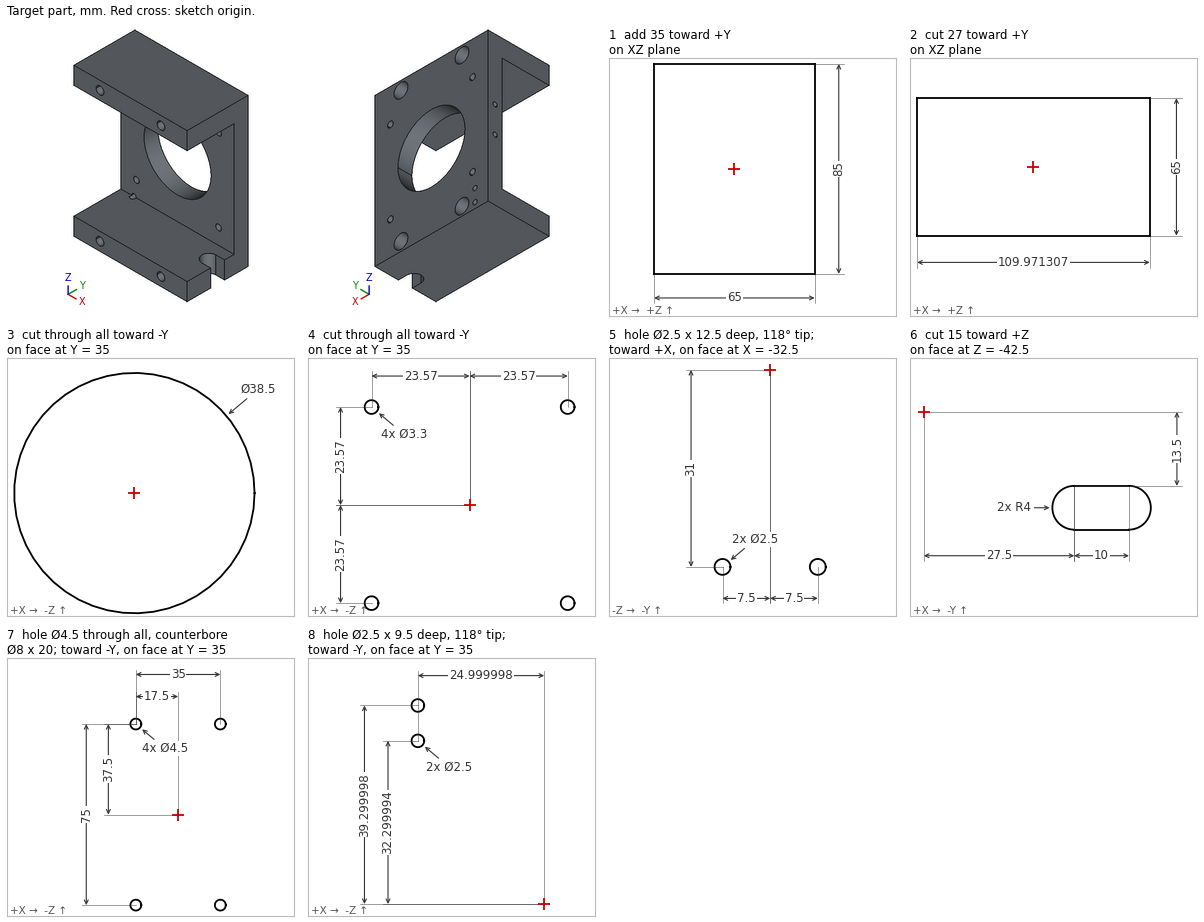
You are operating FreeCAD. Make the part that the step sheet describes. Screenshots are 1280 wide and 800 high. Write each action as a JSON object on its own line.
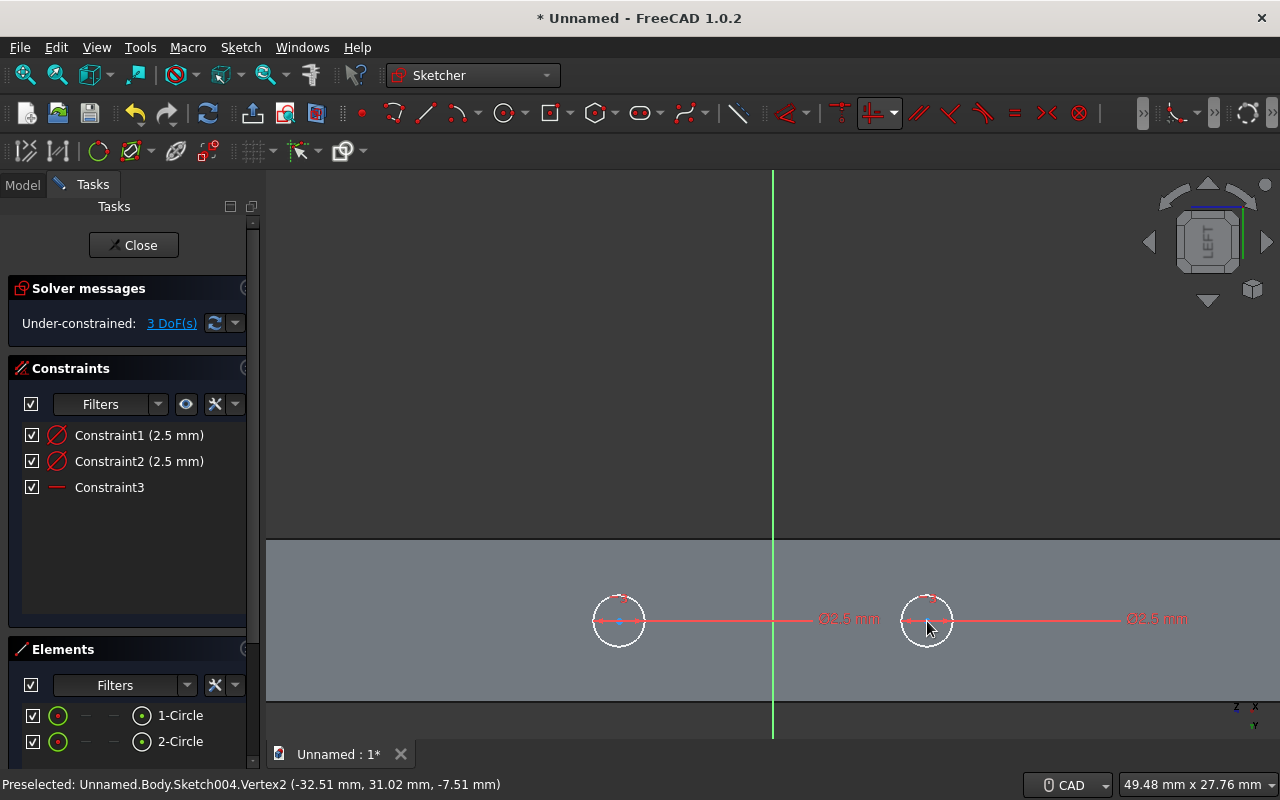
{"action": "left_click", "coordinate": [786, 114]}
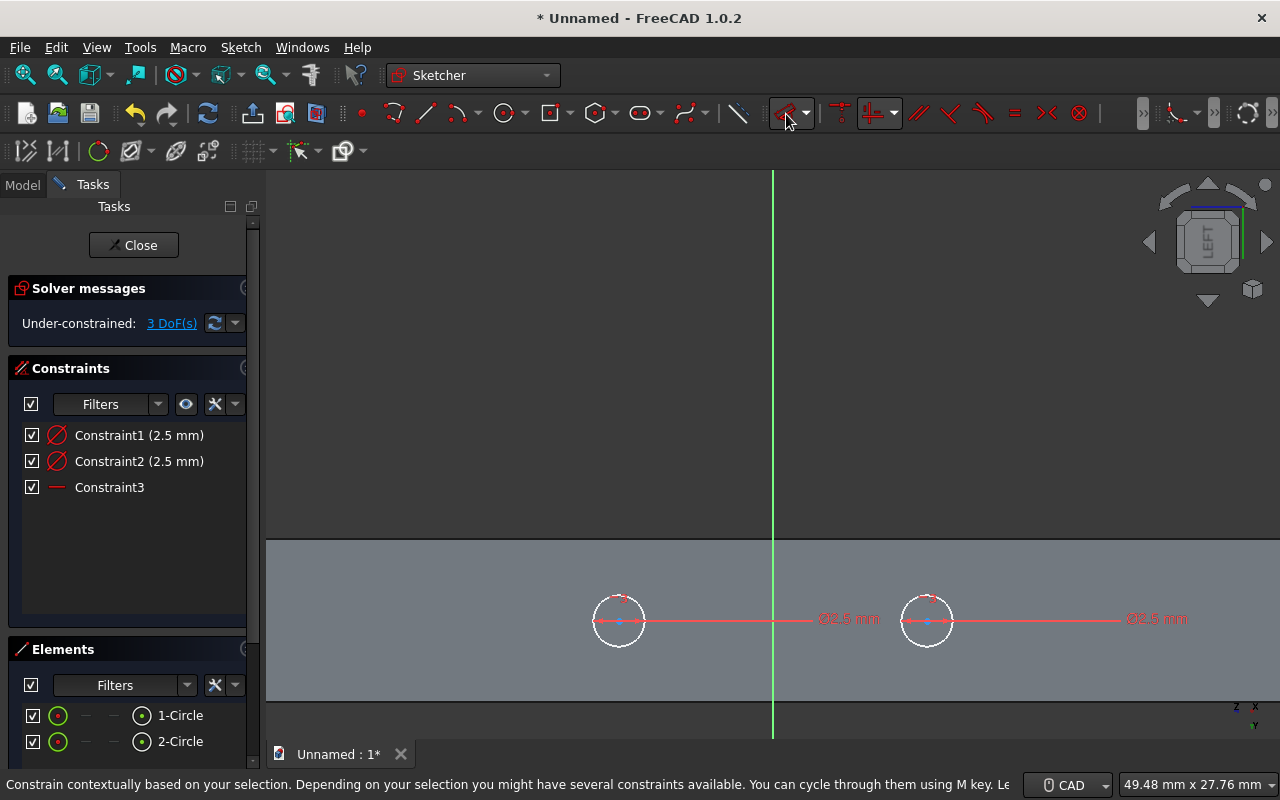
{"action": "left_click", "coordinate": [619, 621]}
{"action": "left_click", "coordinate": [585, 410]}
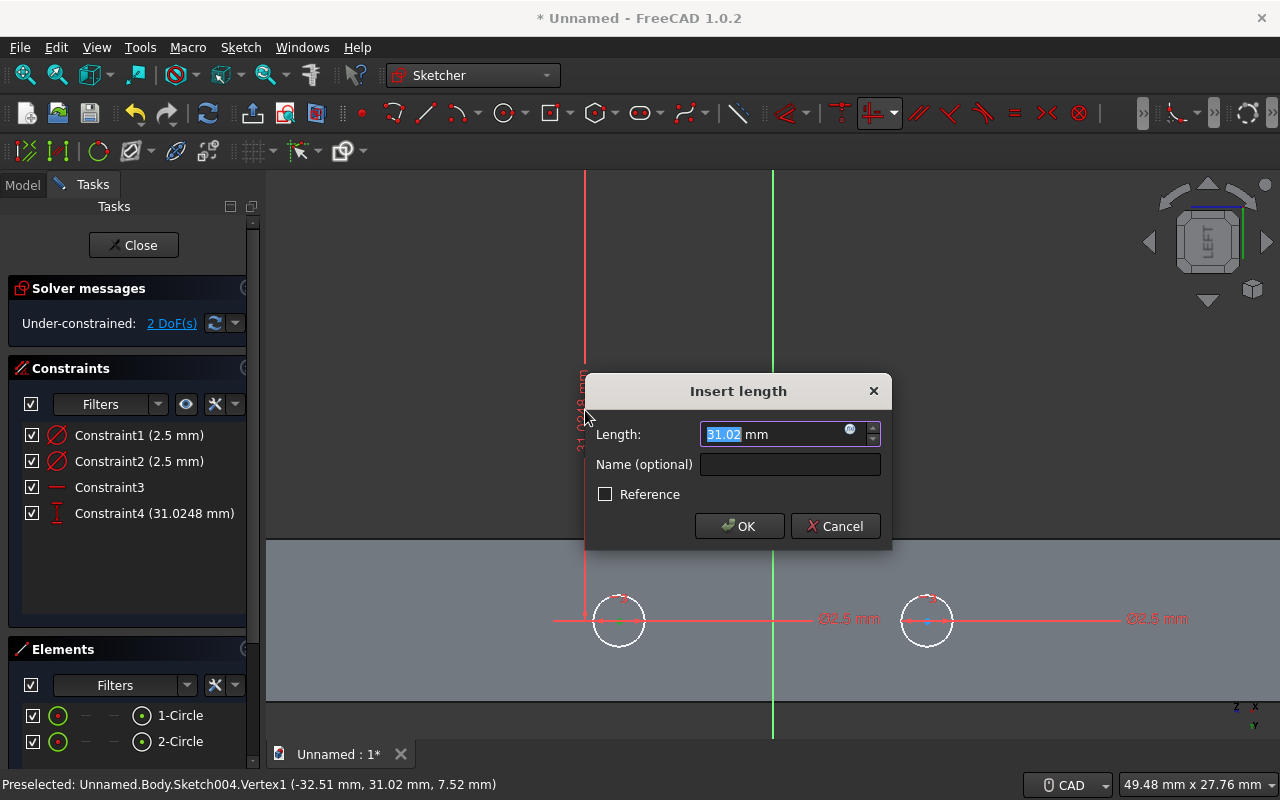
{"action": "type", "text": "31"}
{"action": "key", "text": "Return"}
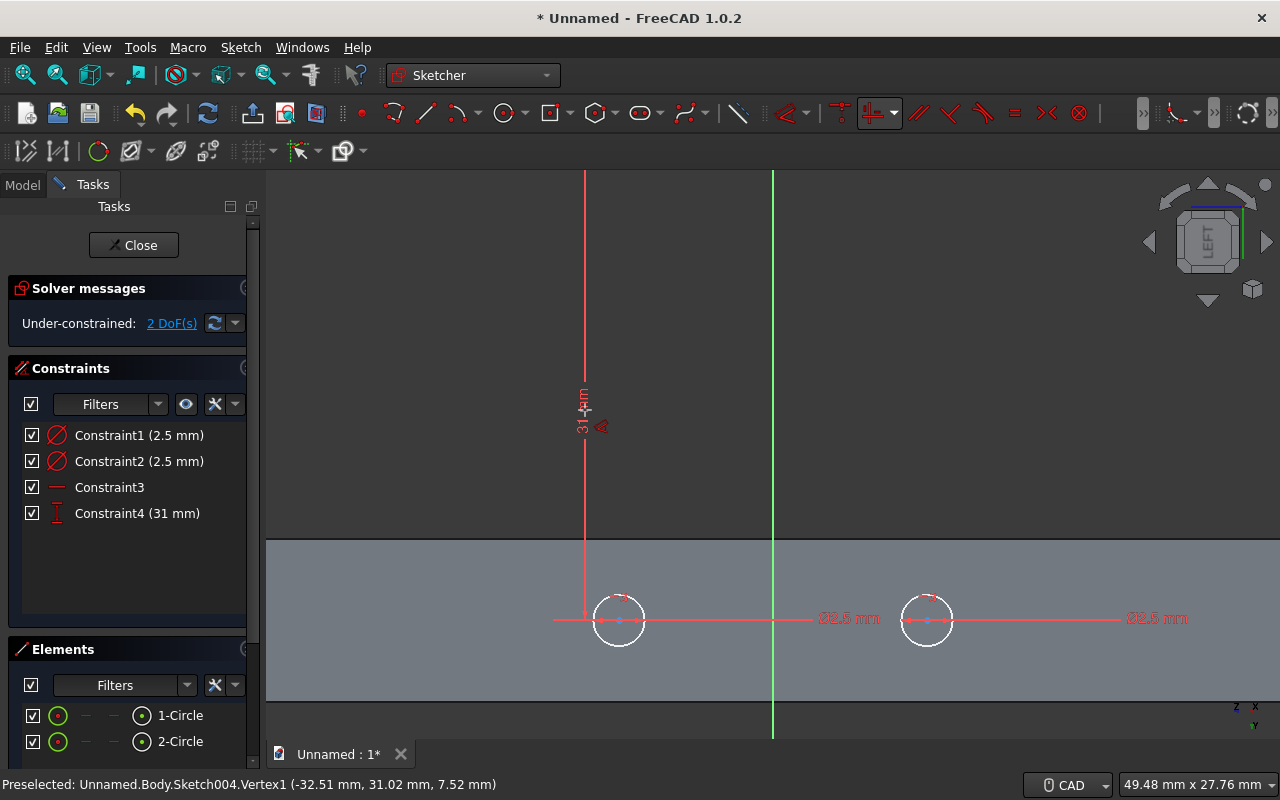
{"action": "left_click", "coordinate": [619, 620]}
{"action": "left_click", "coordinate": [696, 654]}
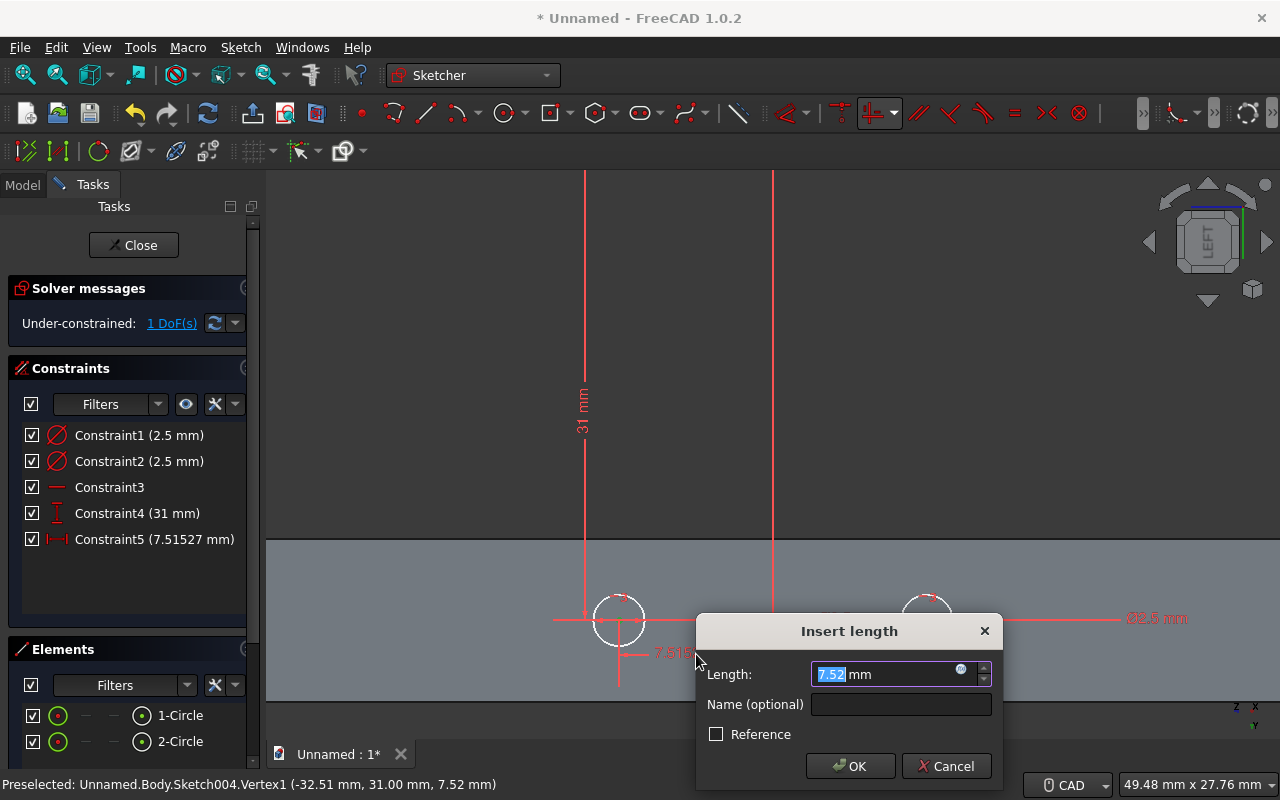
{"action": "type", "text": "7.5"}
{"action": "key", "text": "Return"}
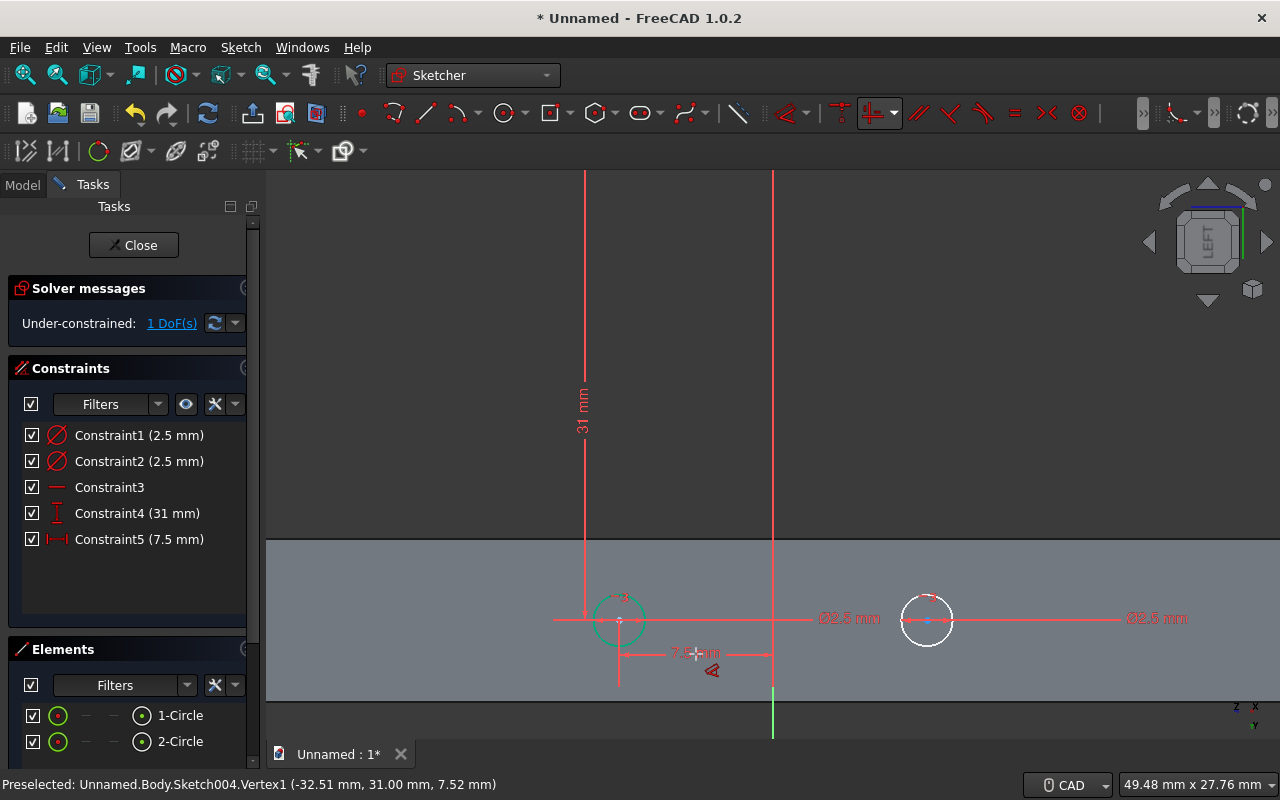
{"action": "left_click", "coordinate": [927, 620]}
{"action": "left_click", "coordinate": [850, 654]}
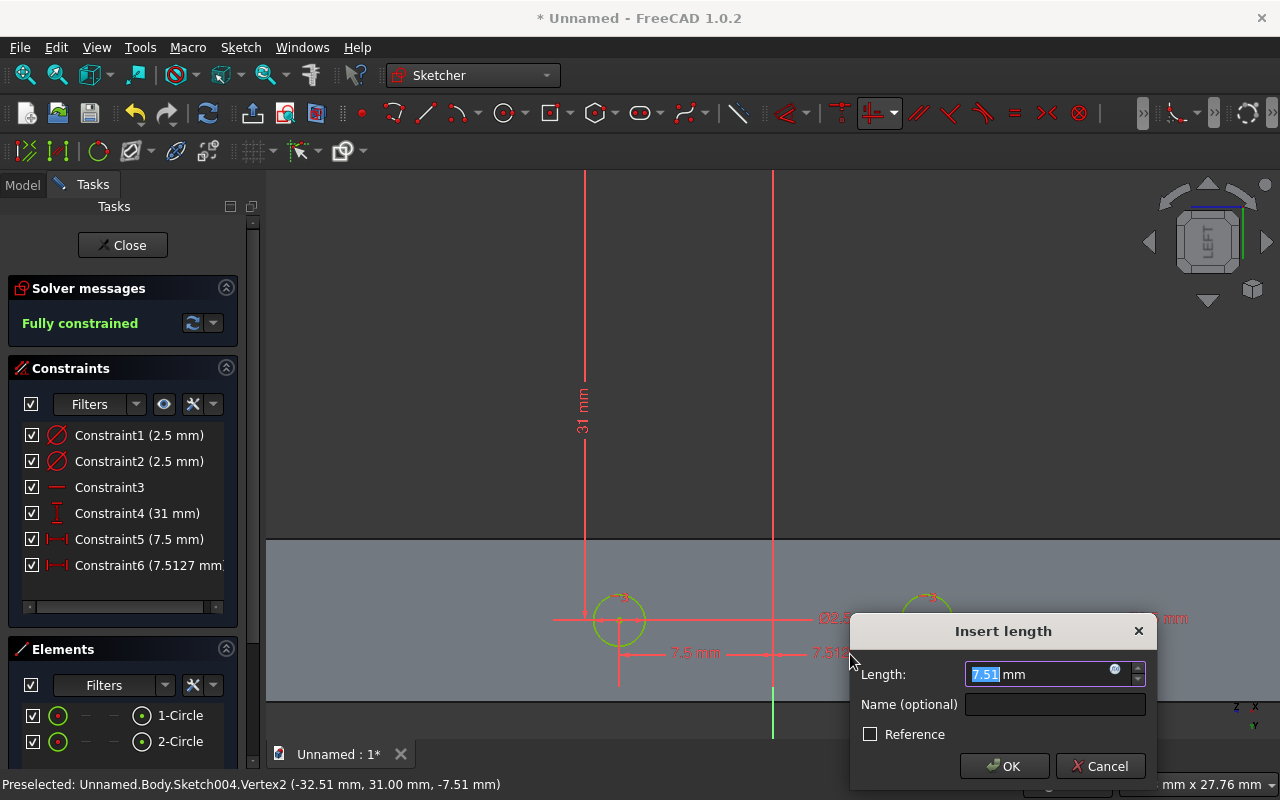
{"action": "type", "text": "7.5"}
{"action": "key", "text": "Return"}
{"action": "key", "text": "Escape"}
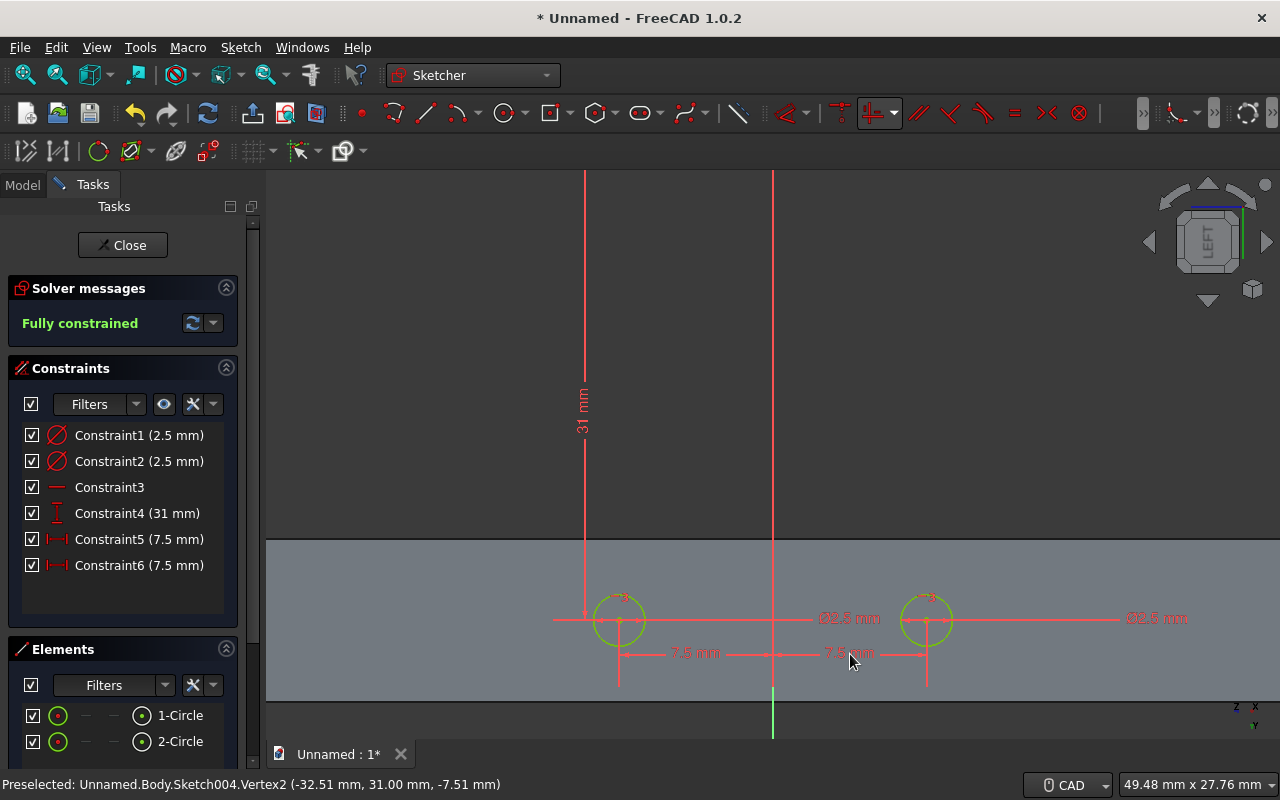
{"action": "left_click", "coordinate": [123, 245]}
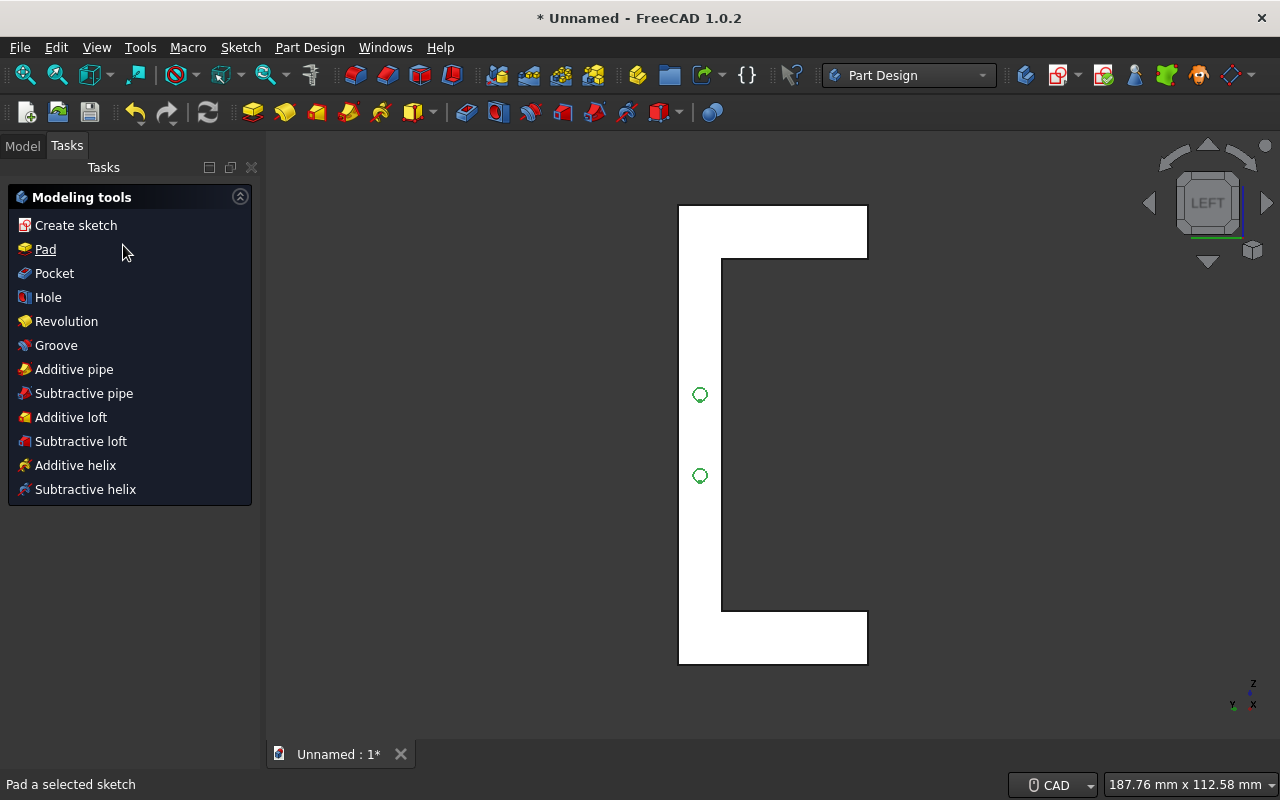
{"action": "left_click", "coordinate": [500, 112]}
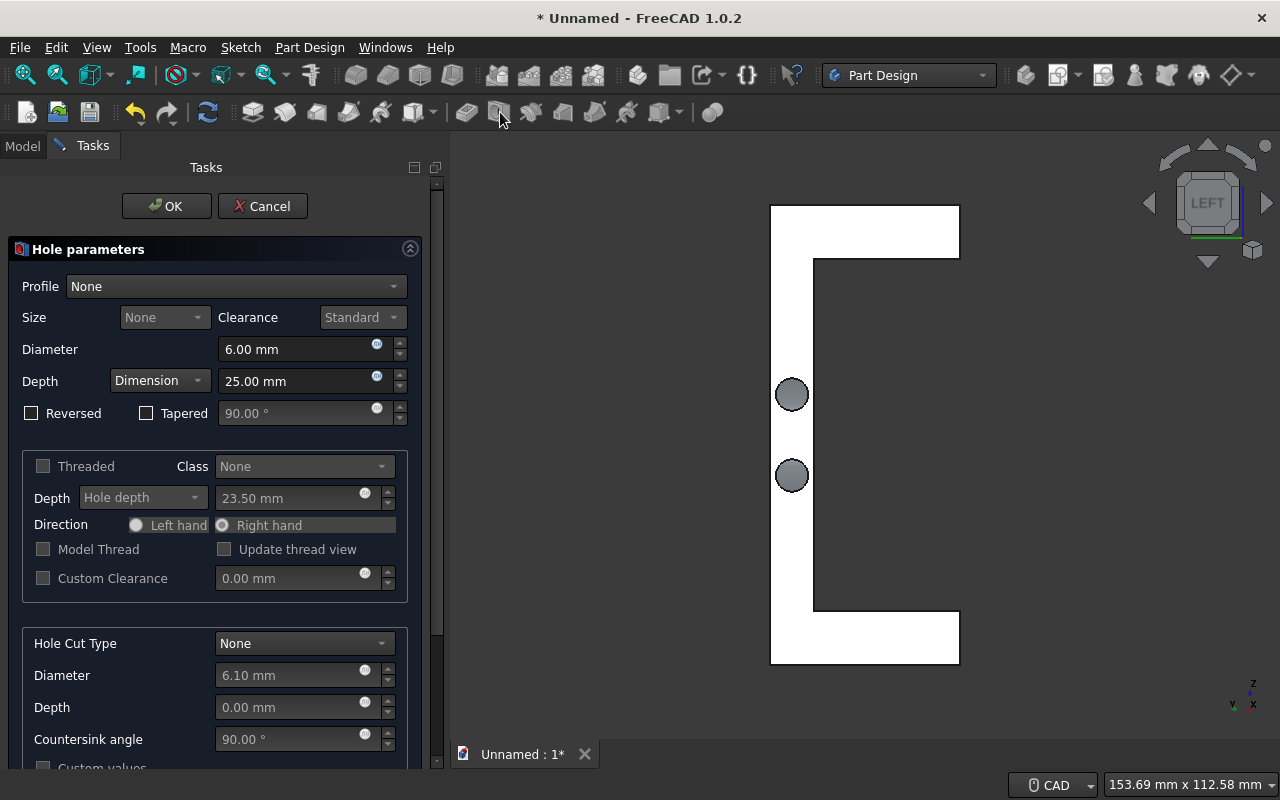
{"action": "triple_click", "coordinate": [305, 349]}